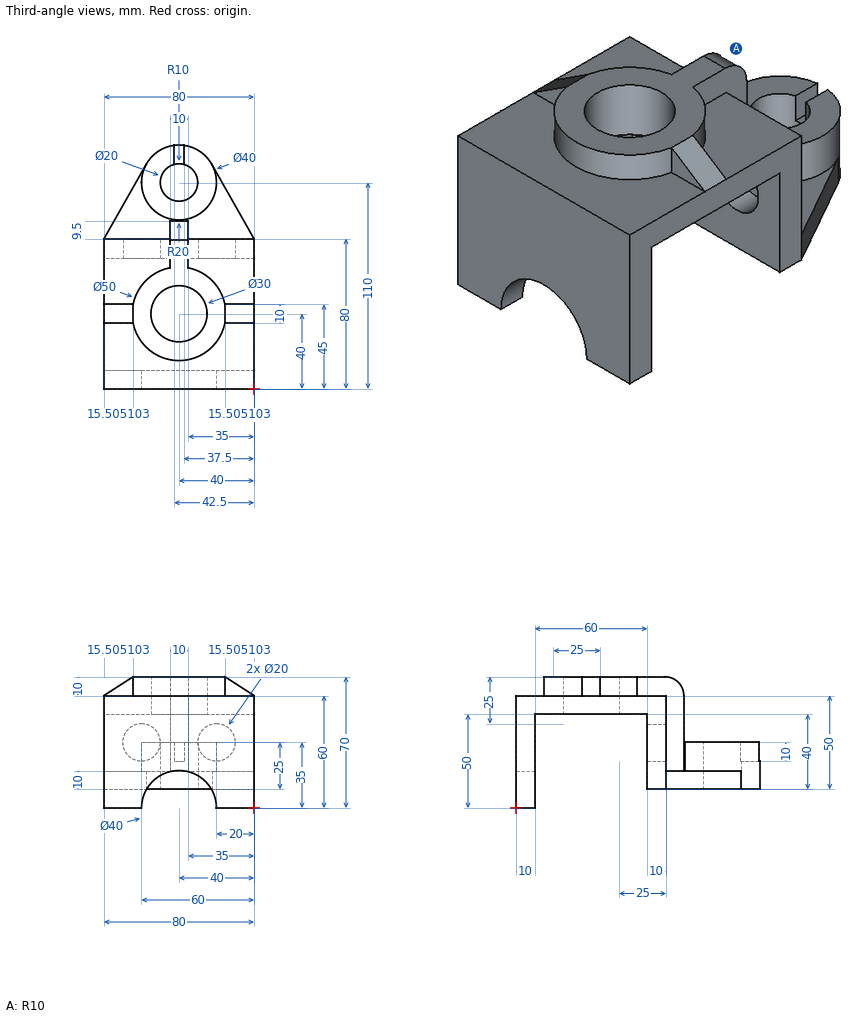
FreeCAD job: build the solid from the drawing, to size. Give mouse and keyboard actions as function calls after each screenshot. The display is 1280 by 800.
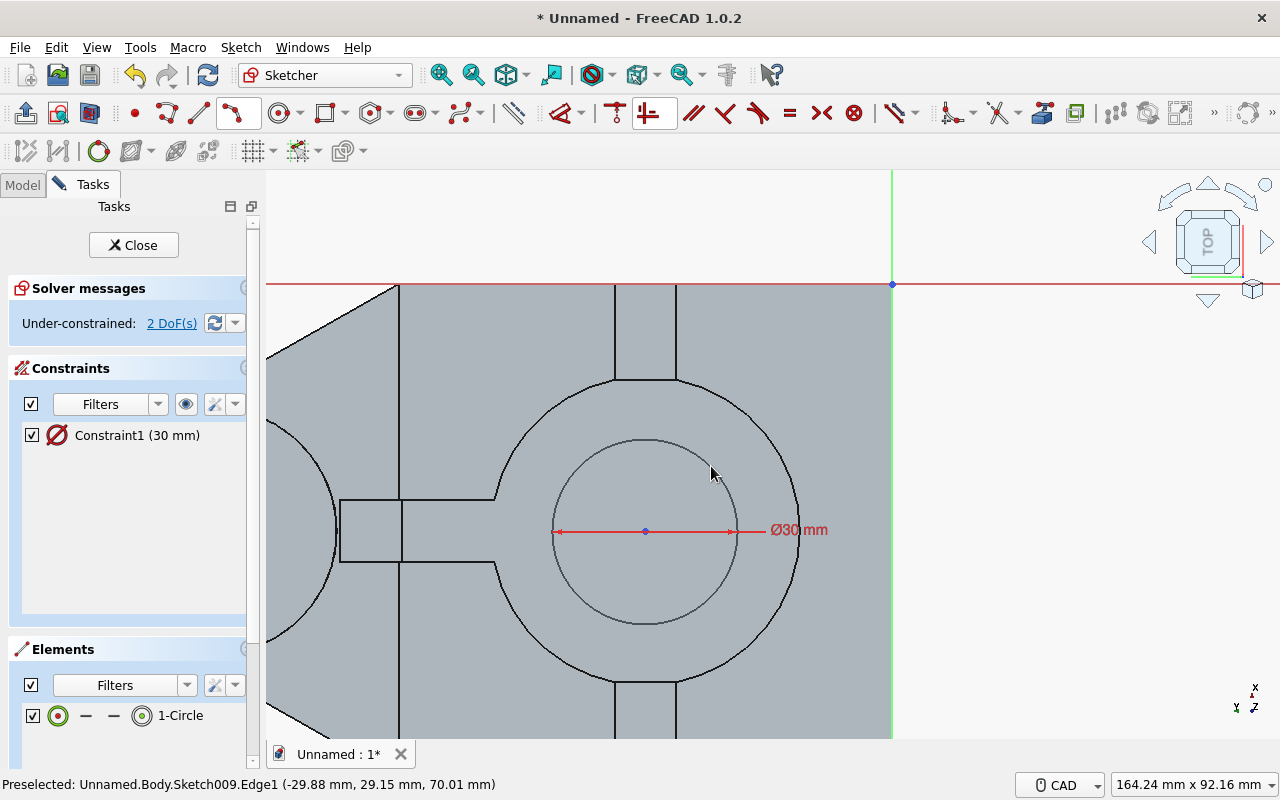
click(560, 114)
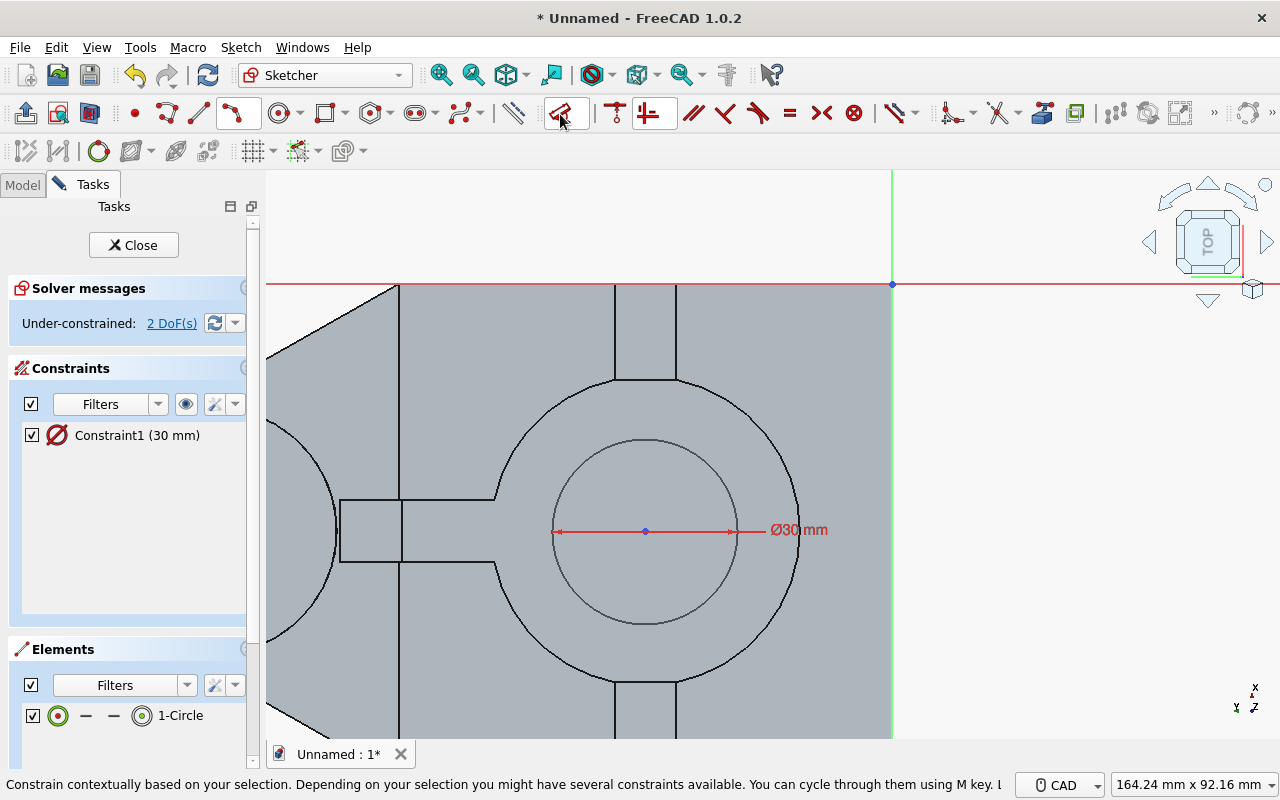
click(645, 532)
click(769, 250)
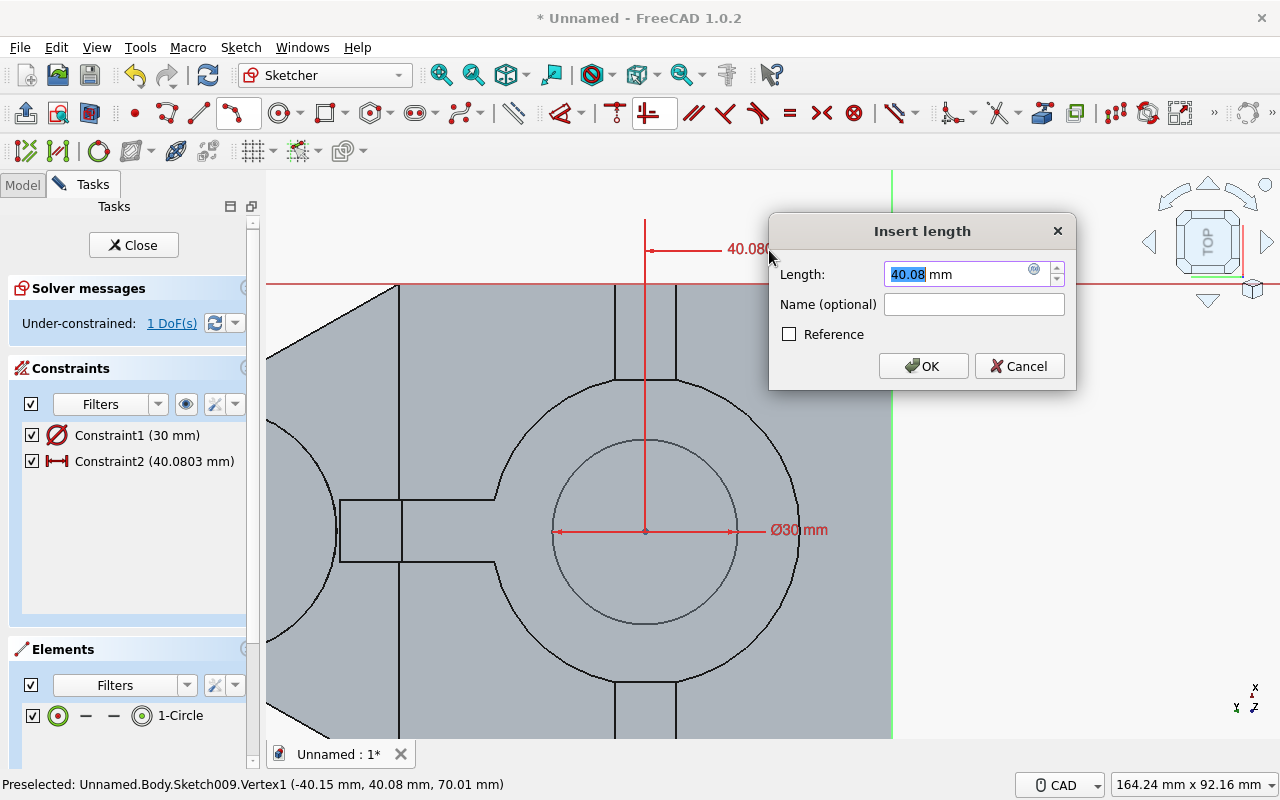
text(40)
key(Return)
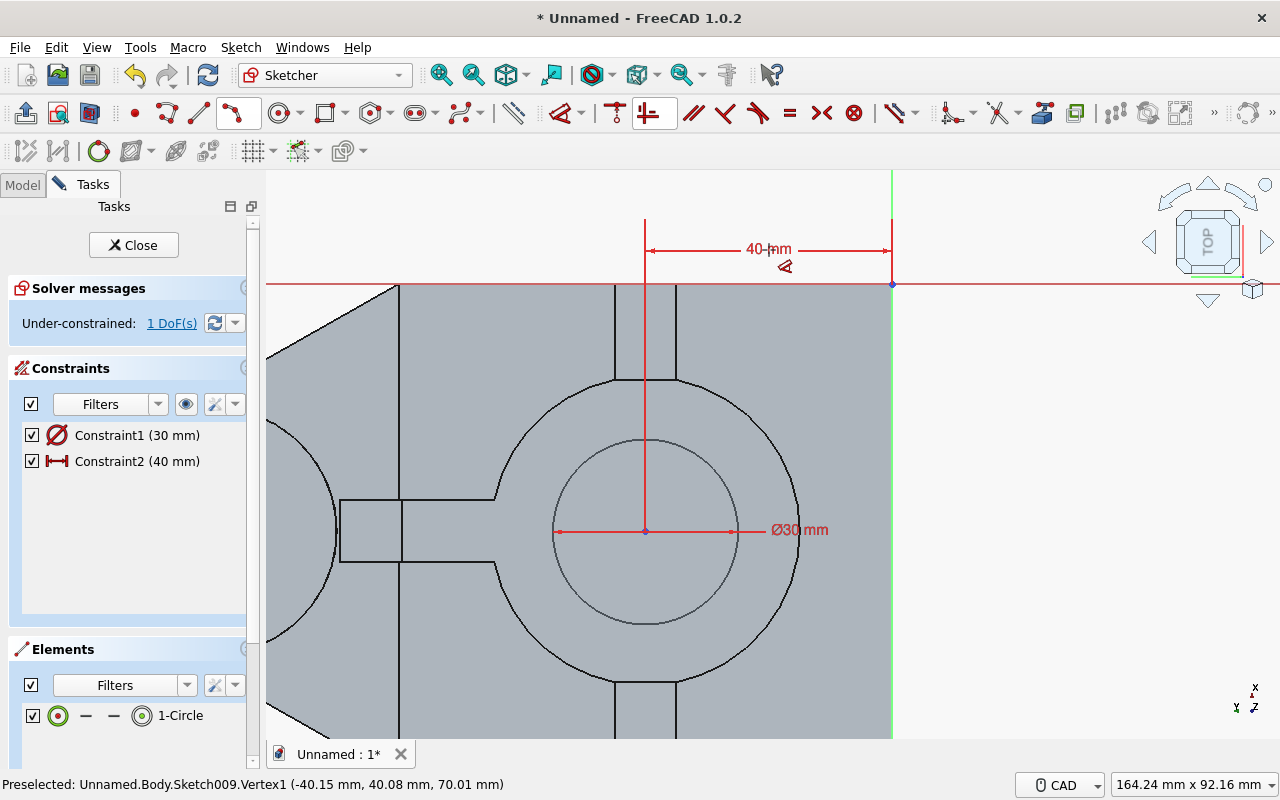
click(645, 532)
click(926, 408)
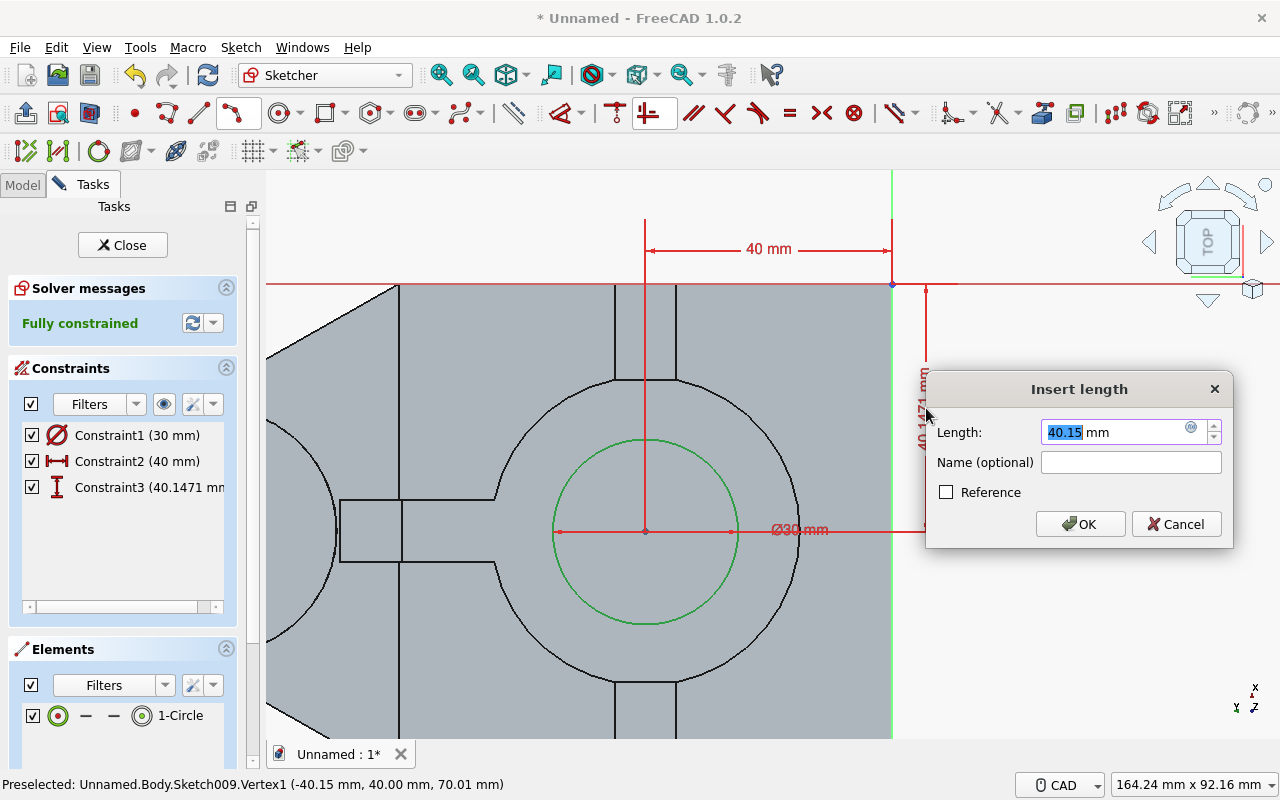
text(40)
key(Return)
key(Escape)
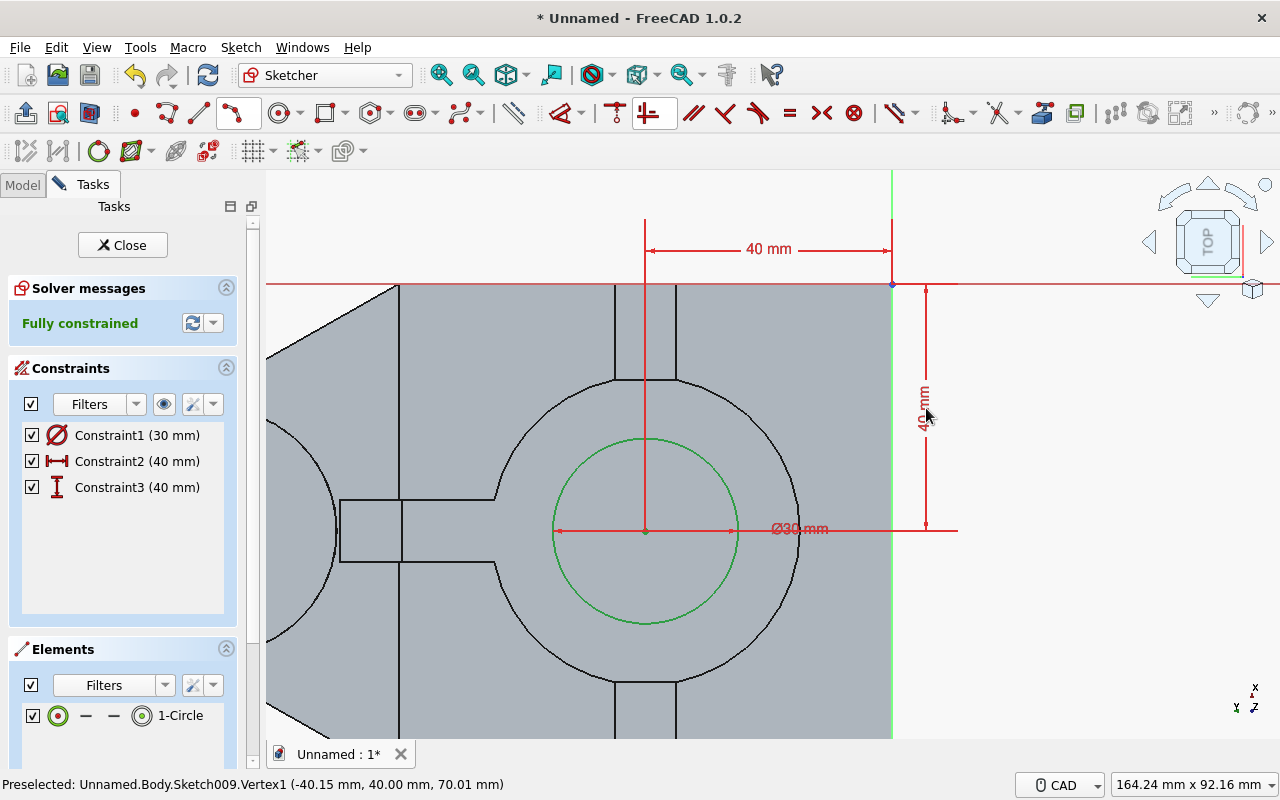
click(123, 245)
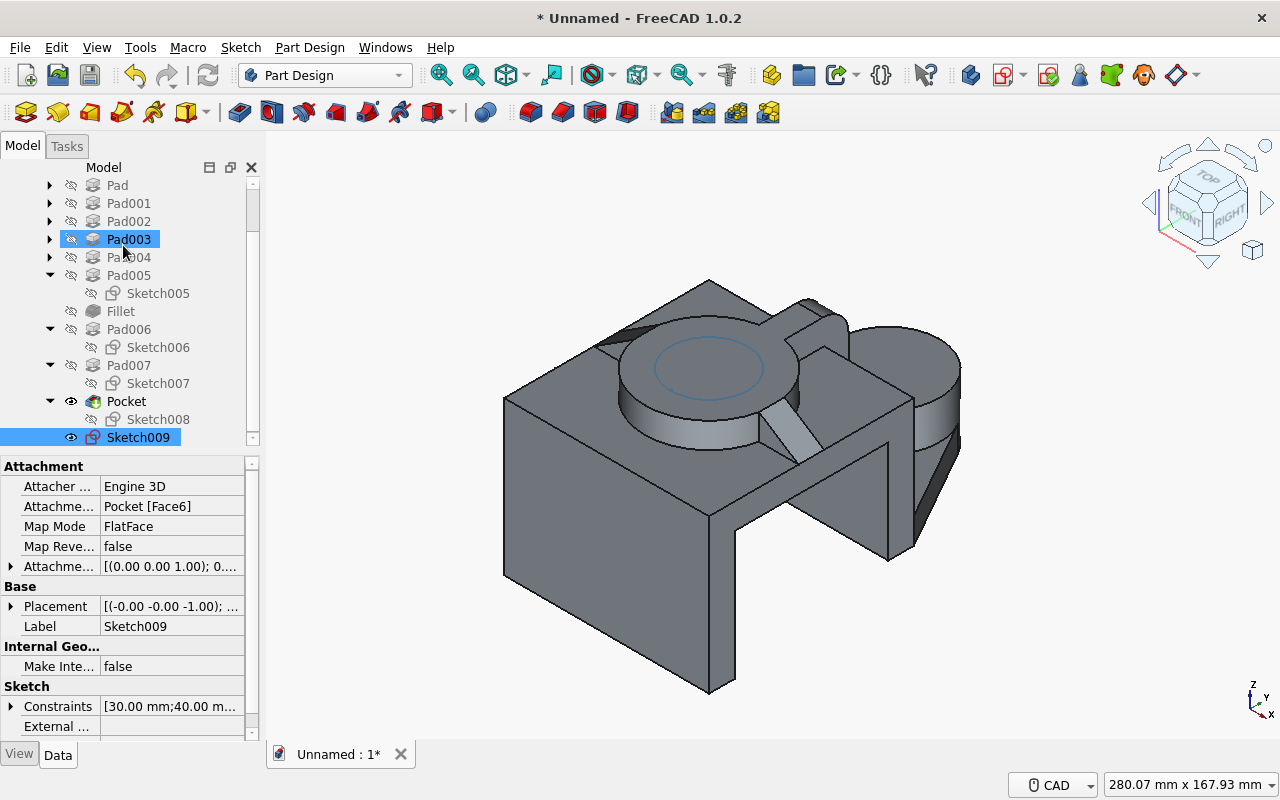
click(240, 112)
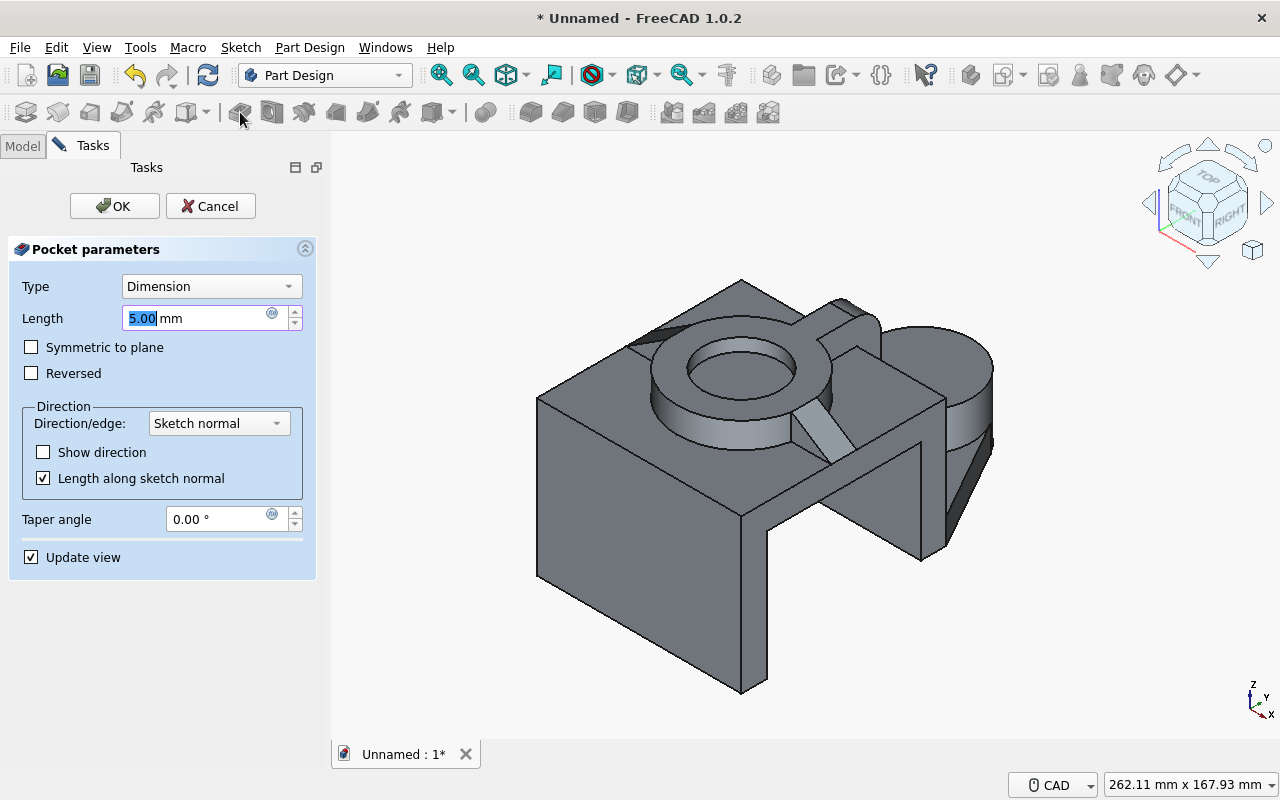
text(25)
key(Tab)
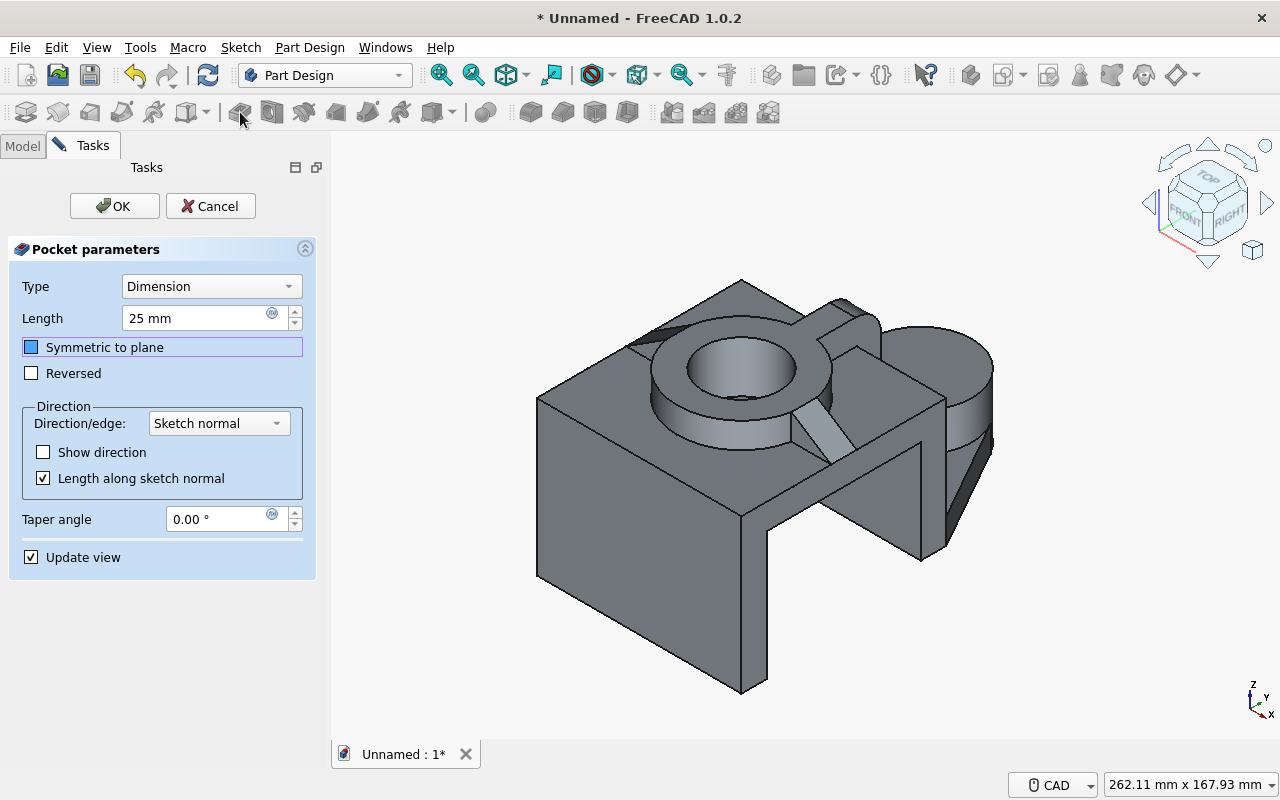
click(115, 206)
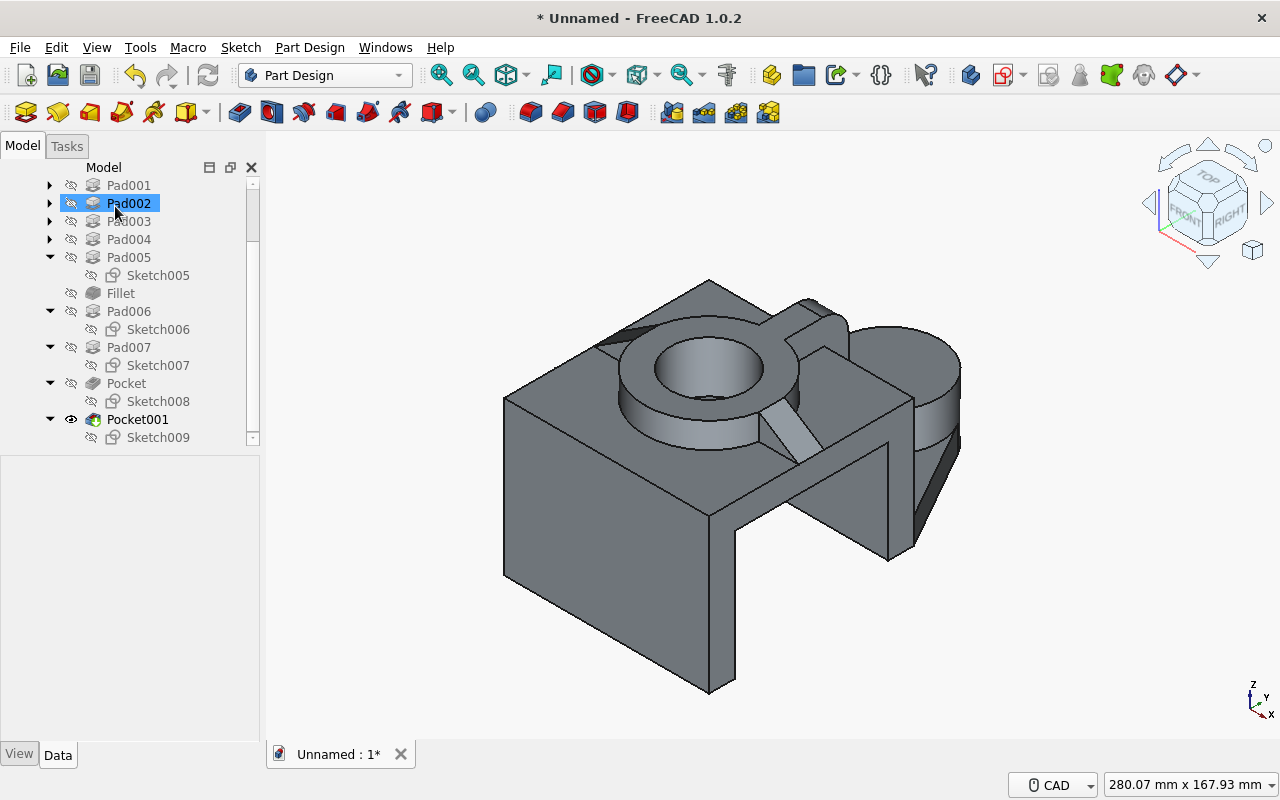
key(4)